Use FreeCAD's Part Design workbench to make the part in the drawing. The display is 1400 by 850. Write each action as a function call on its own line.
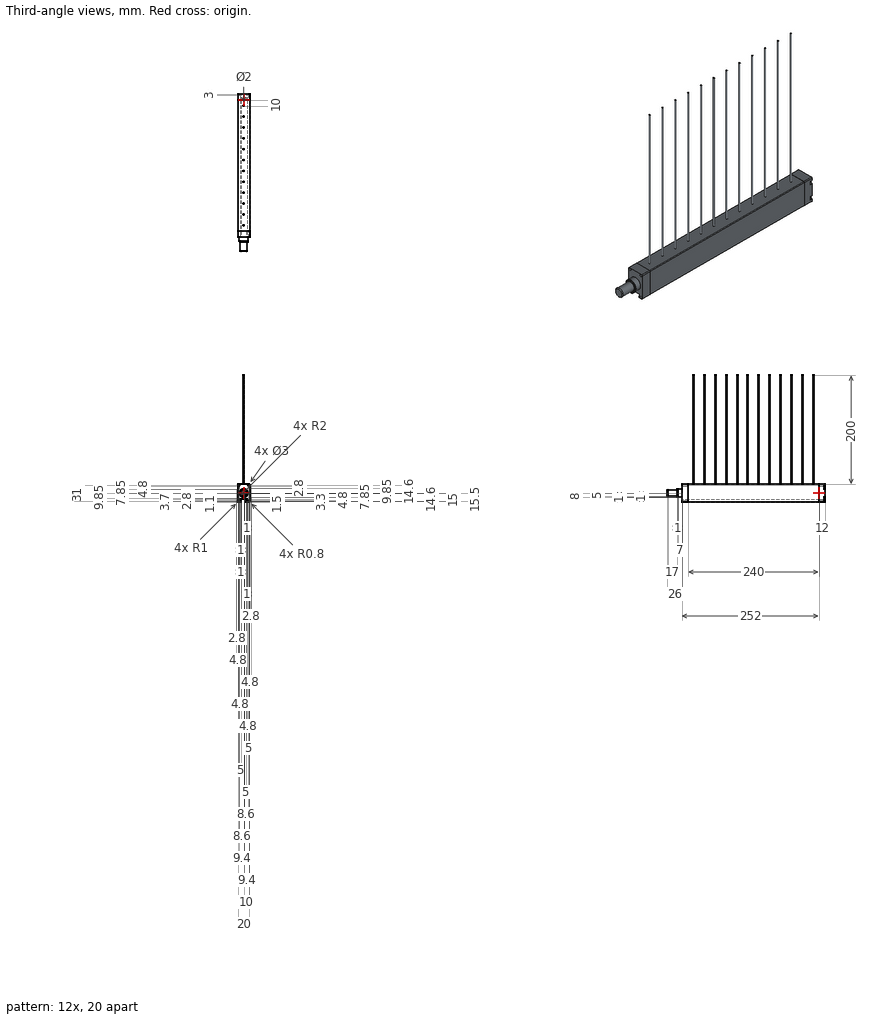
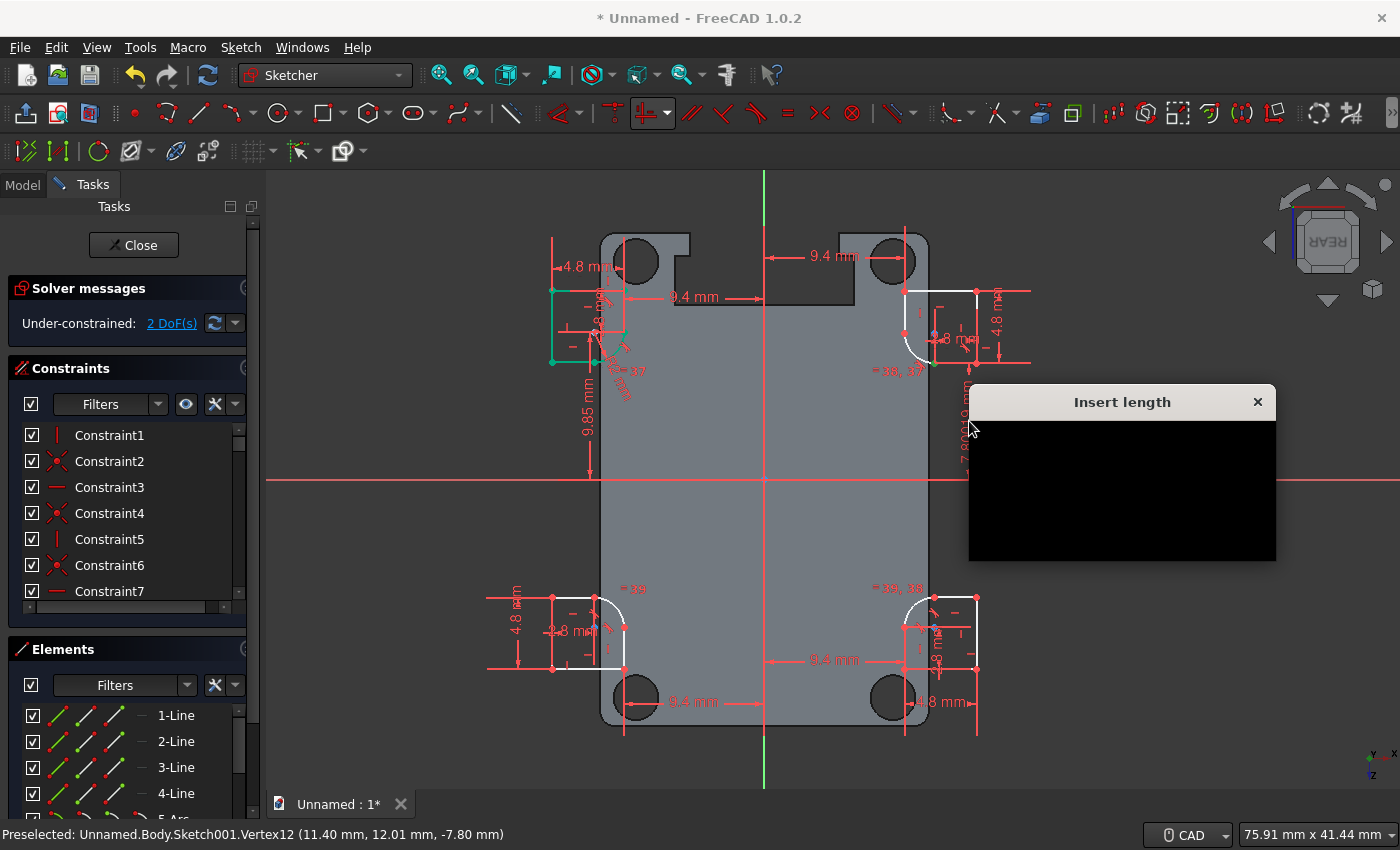
text(7.85)
key(Return)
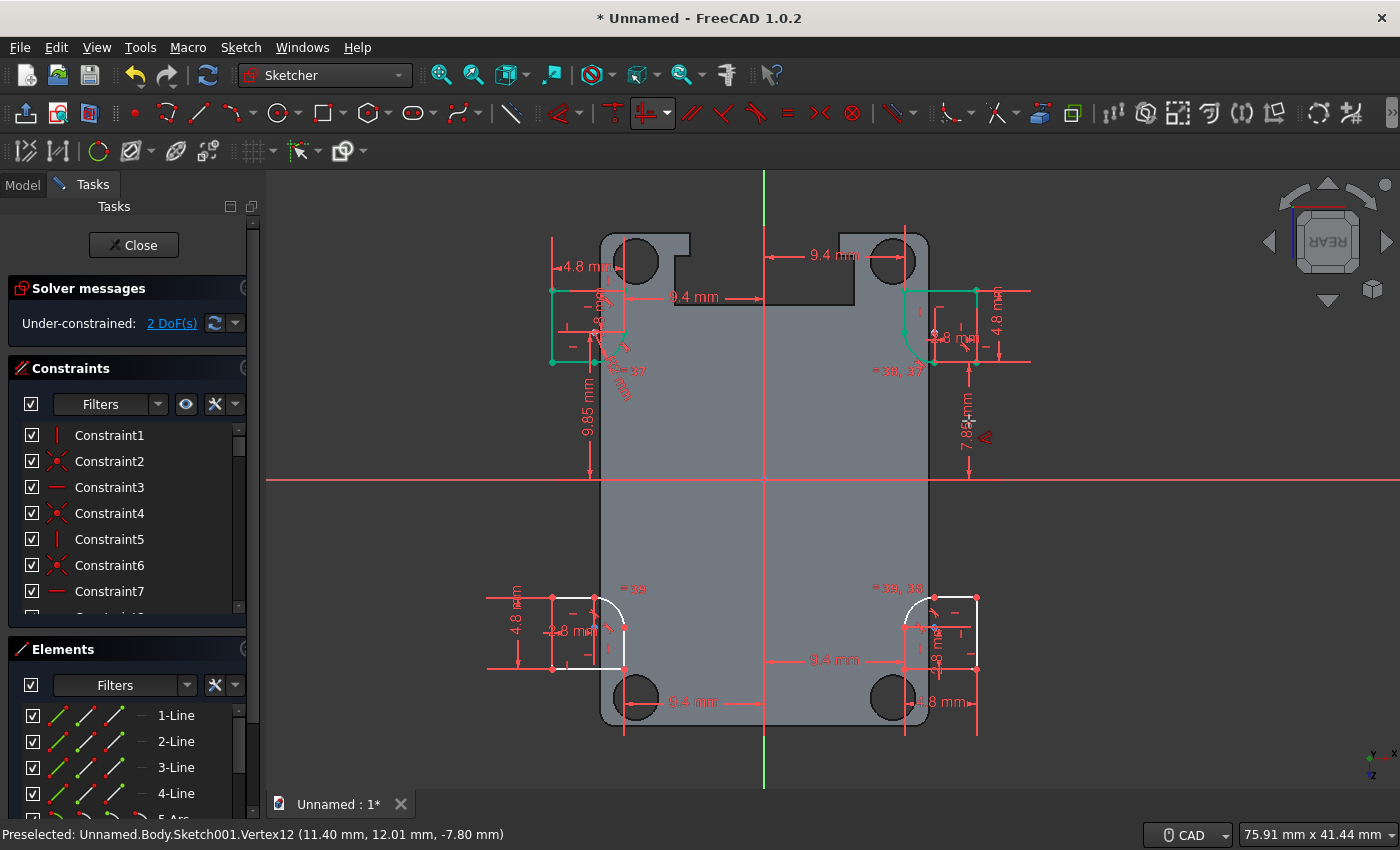
click(905, 627)
click(939, 553)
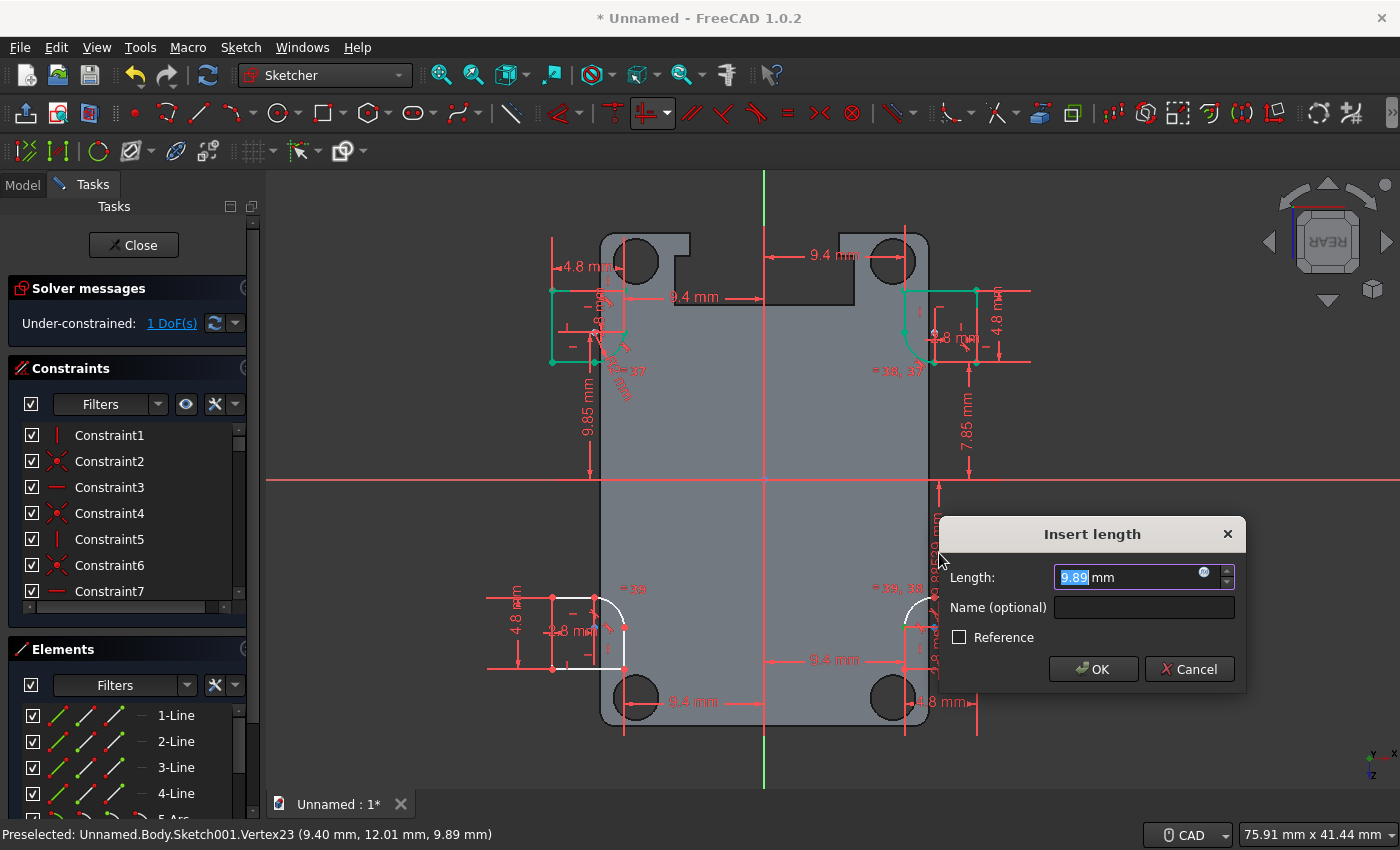
text(9.85)
key(Return)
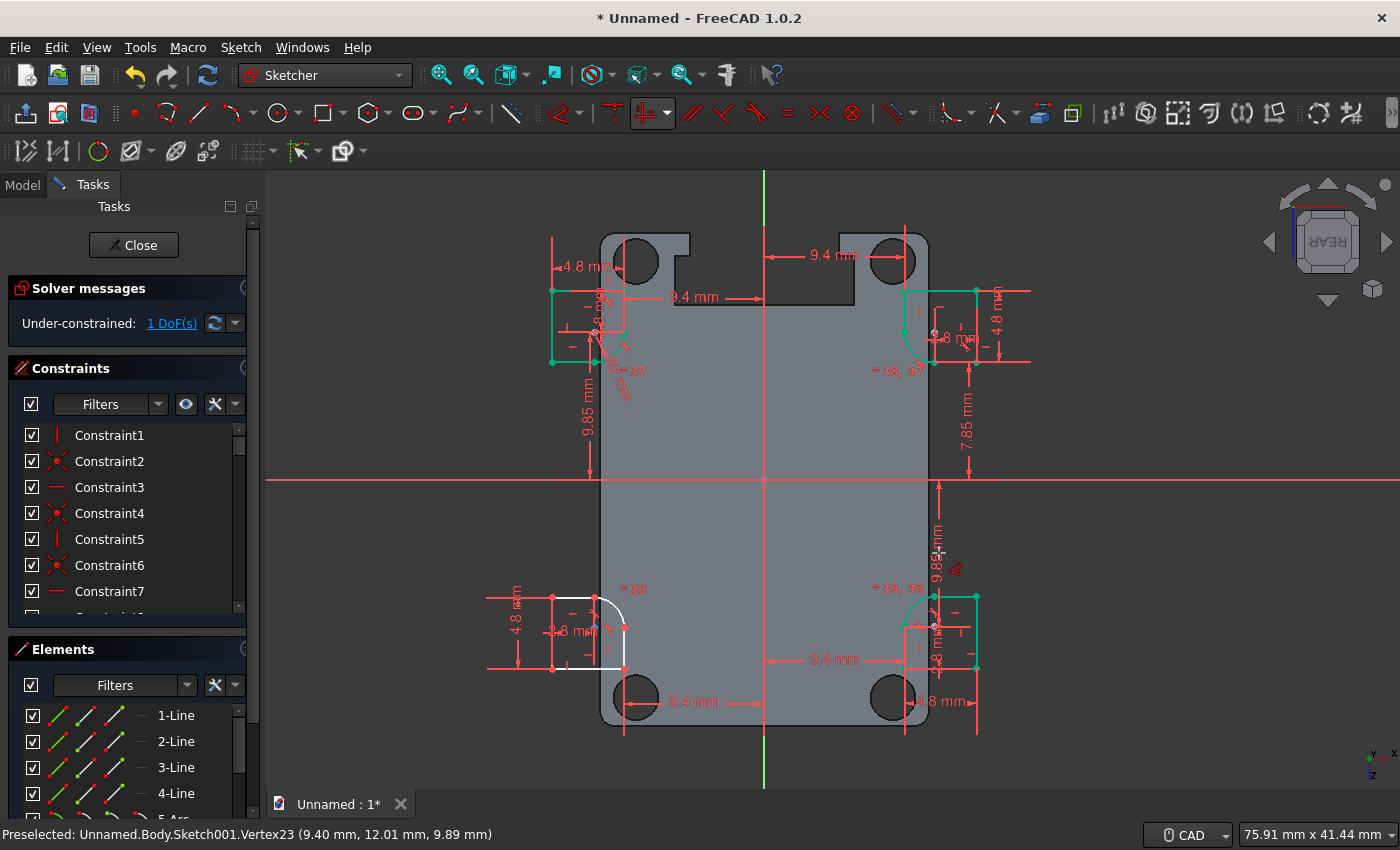
click(594, 598)
click(560, 539)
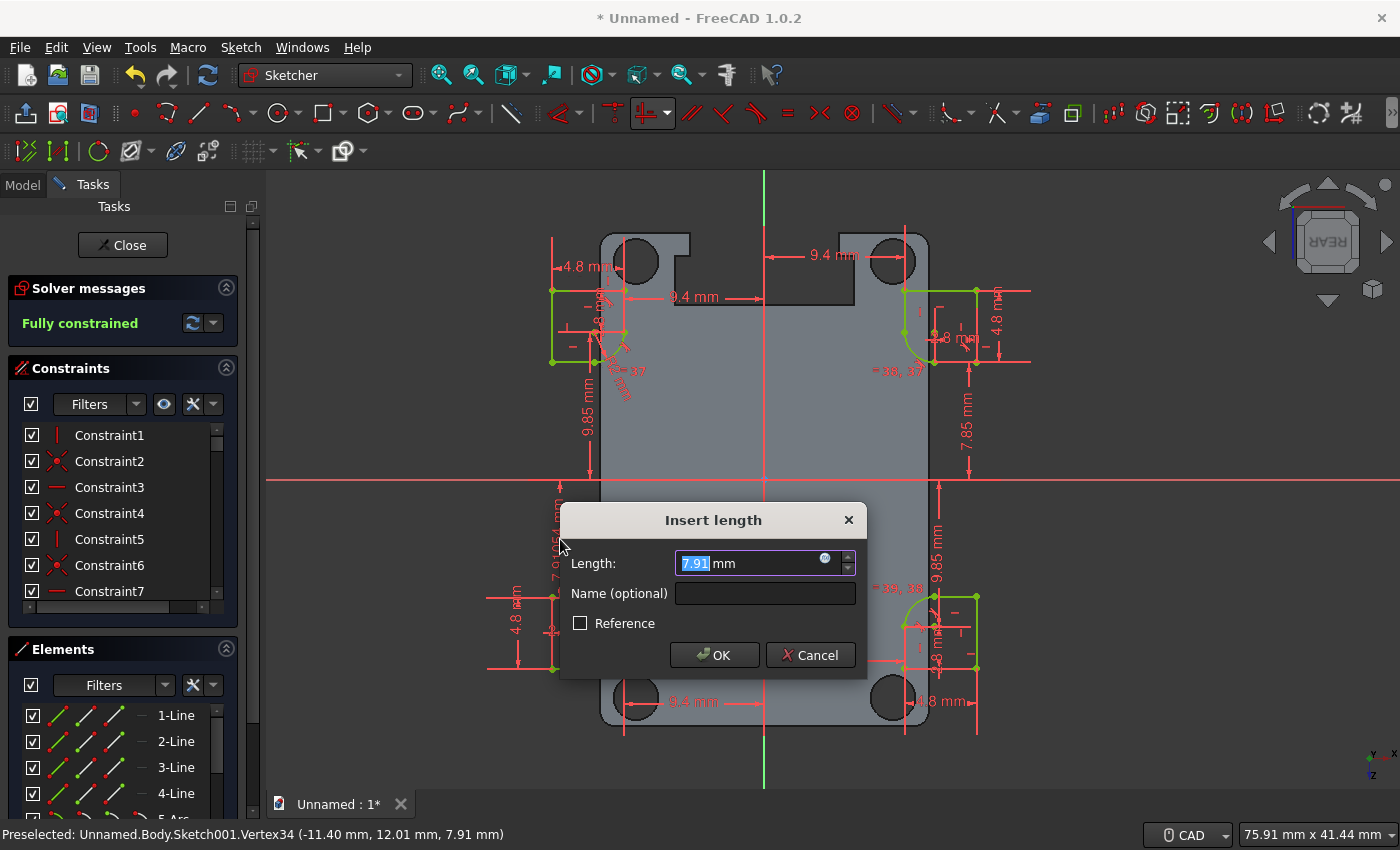
text(7.85)
key(Return)
key(Escape)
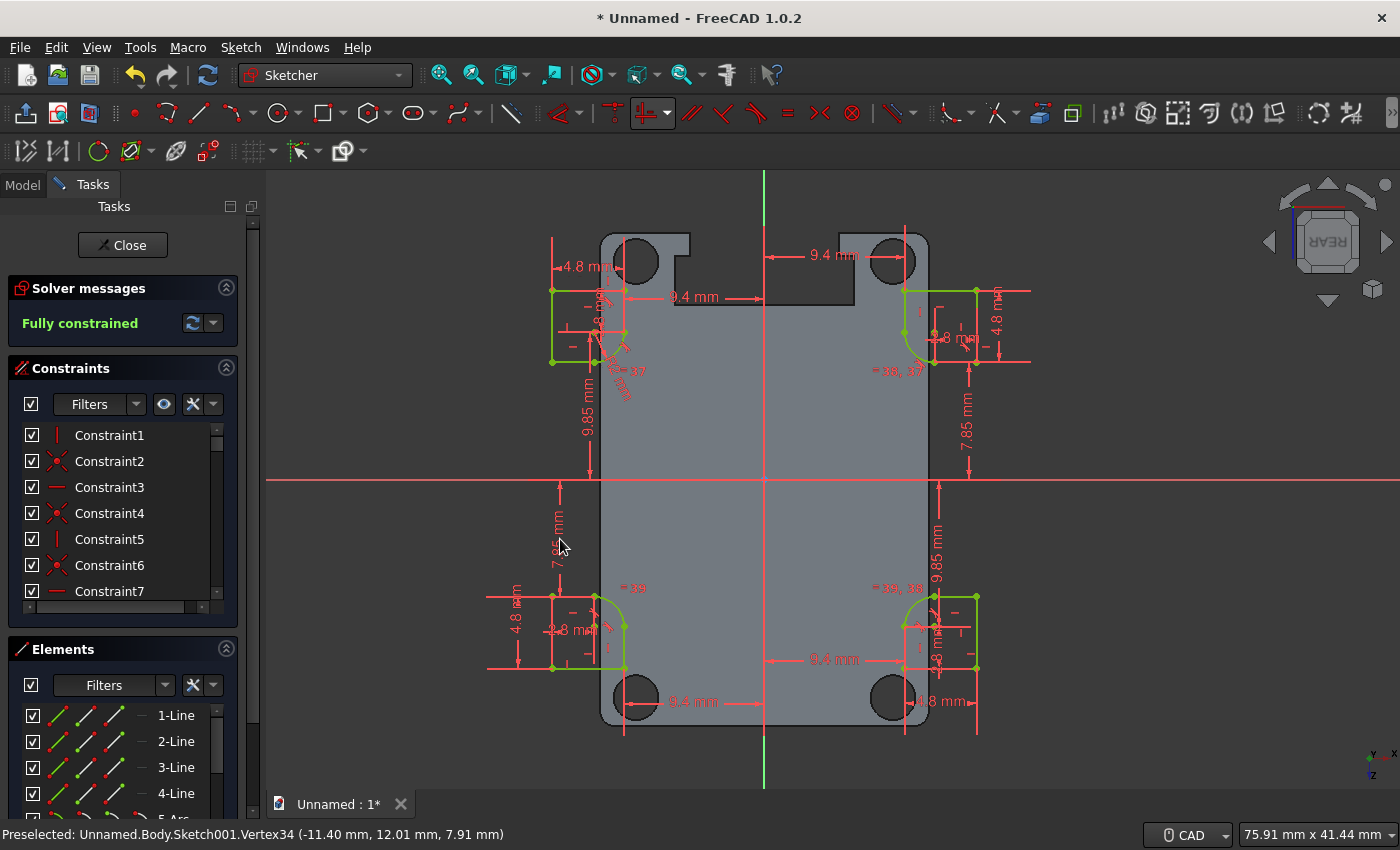
click(123, 245)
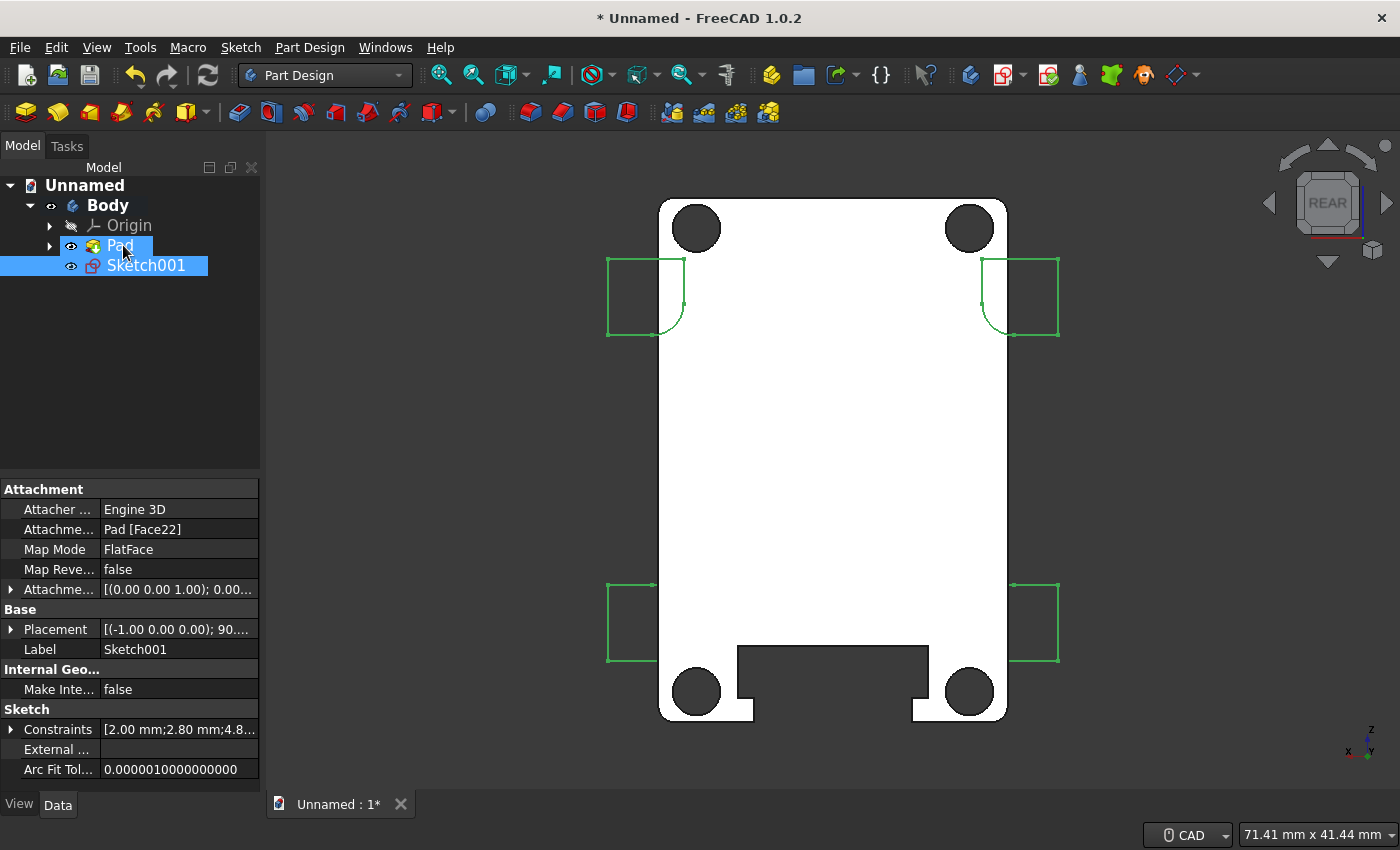
click(240, 112)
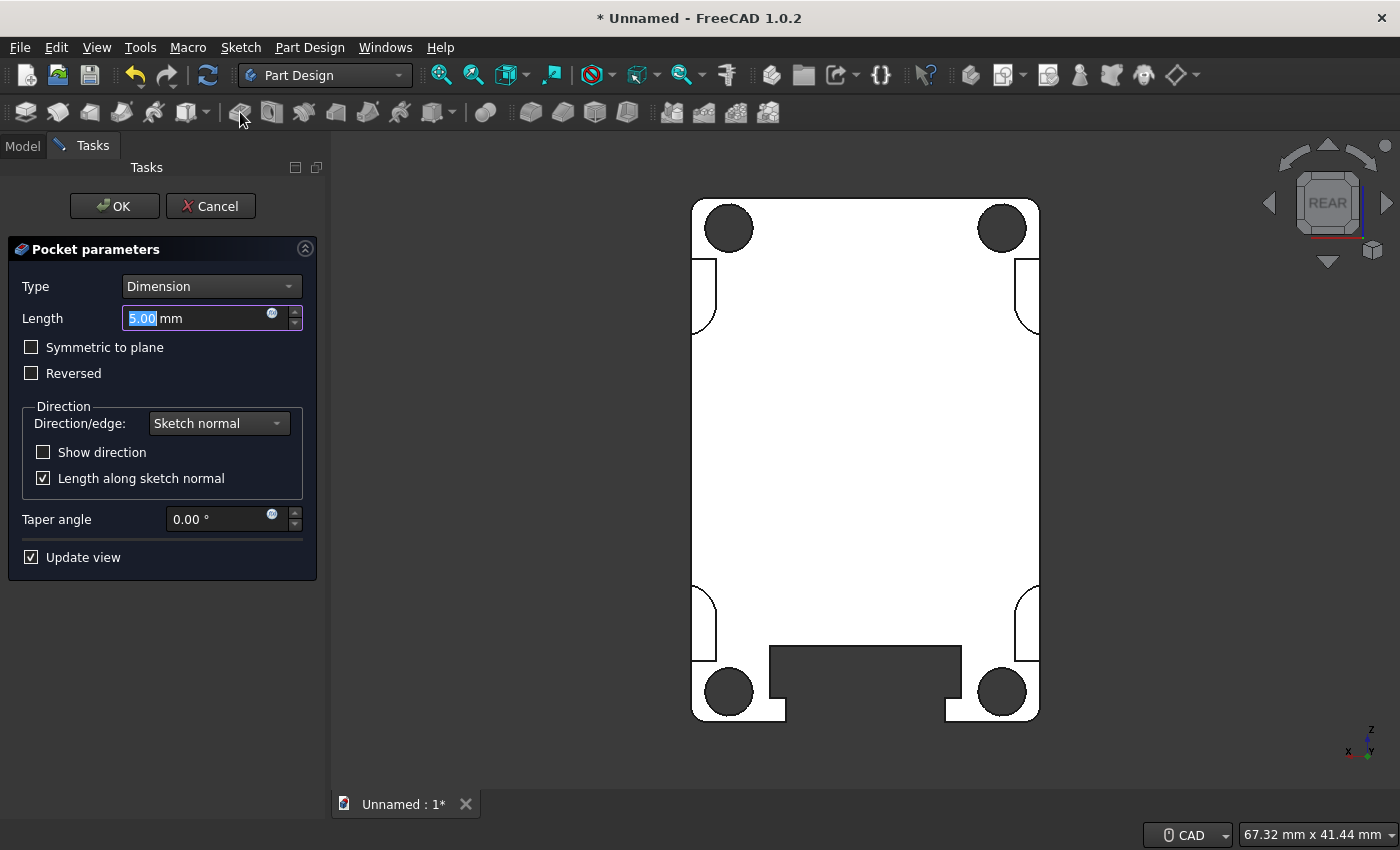
text(3)
key(Tab)